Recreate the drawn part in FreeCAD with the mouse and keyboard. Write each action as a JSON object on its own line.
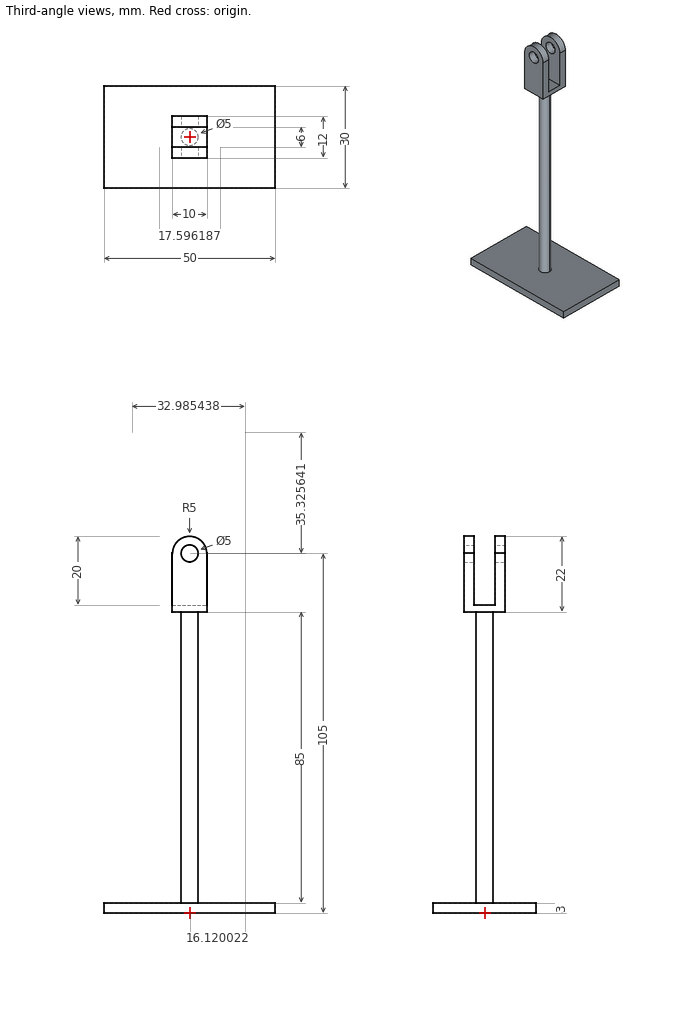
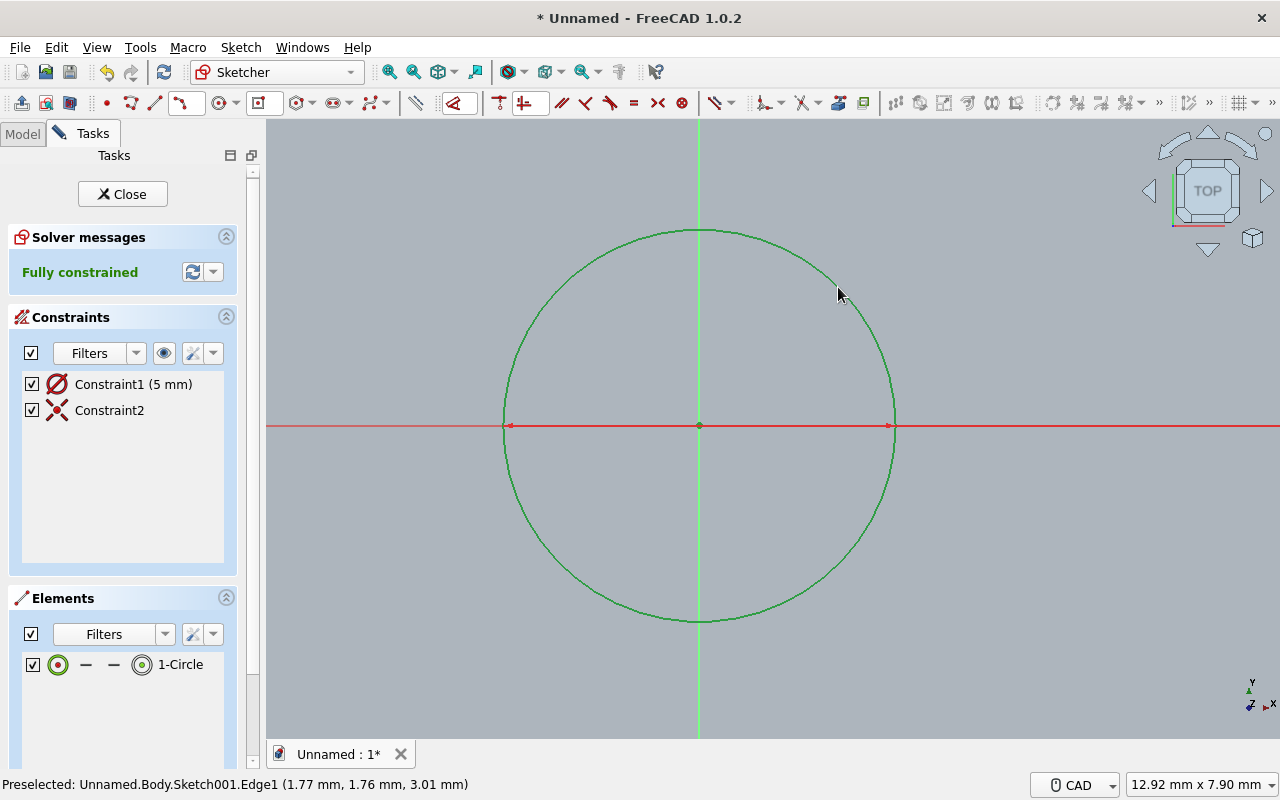
{"action": "left_click", "coordinate": [123, 194]}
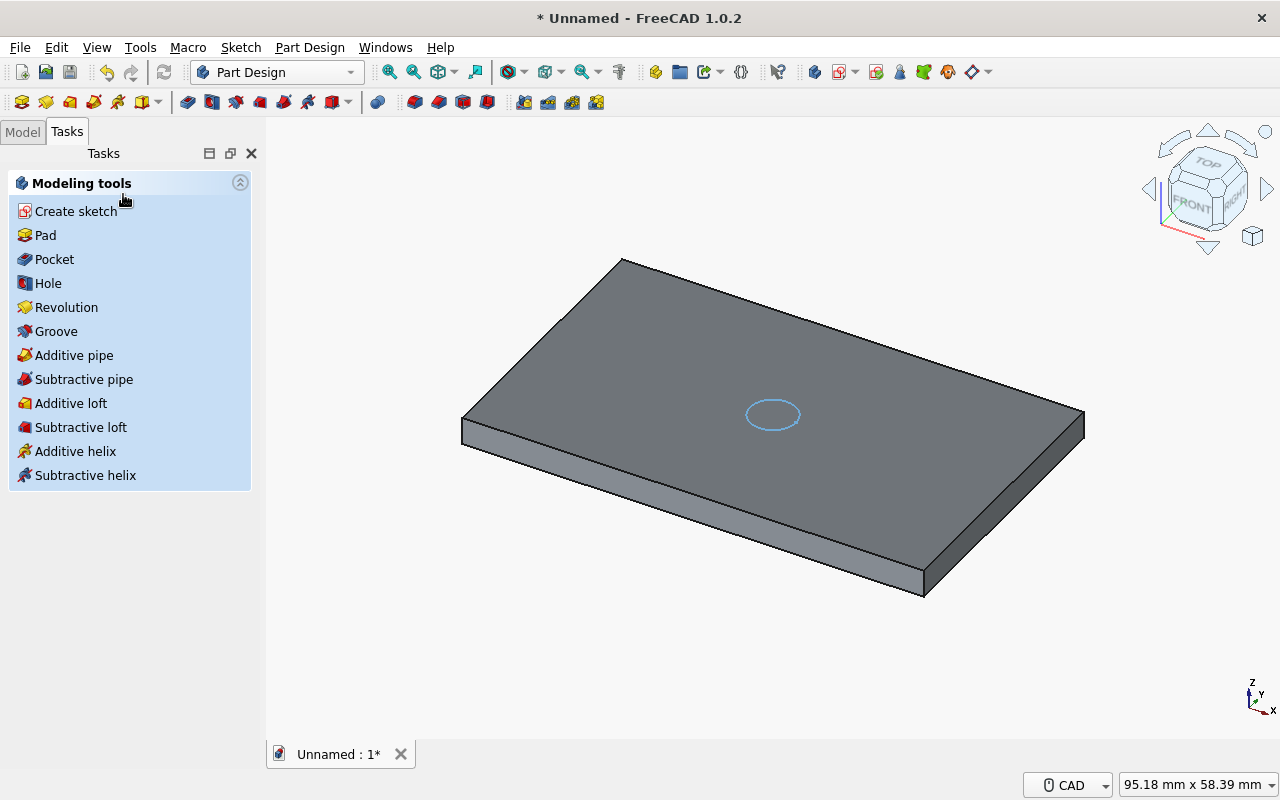
{"action": "left_click", "coordinate": [22, 102]}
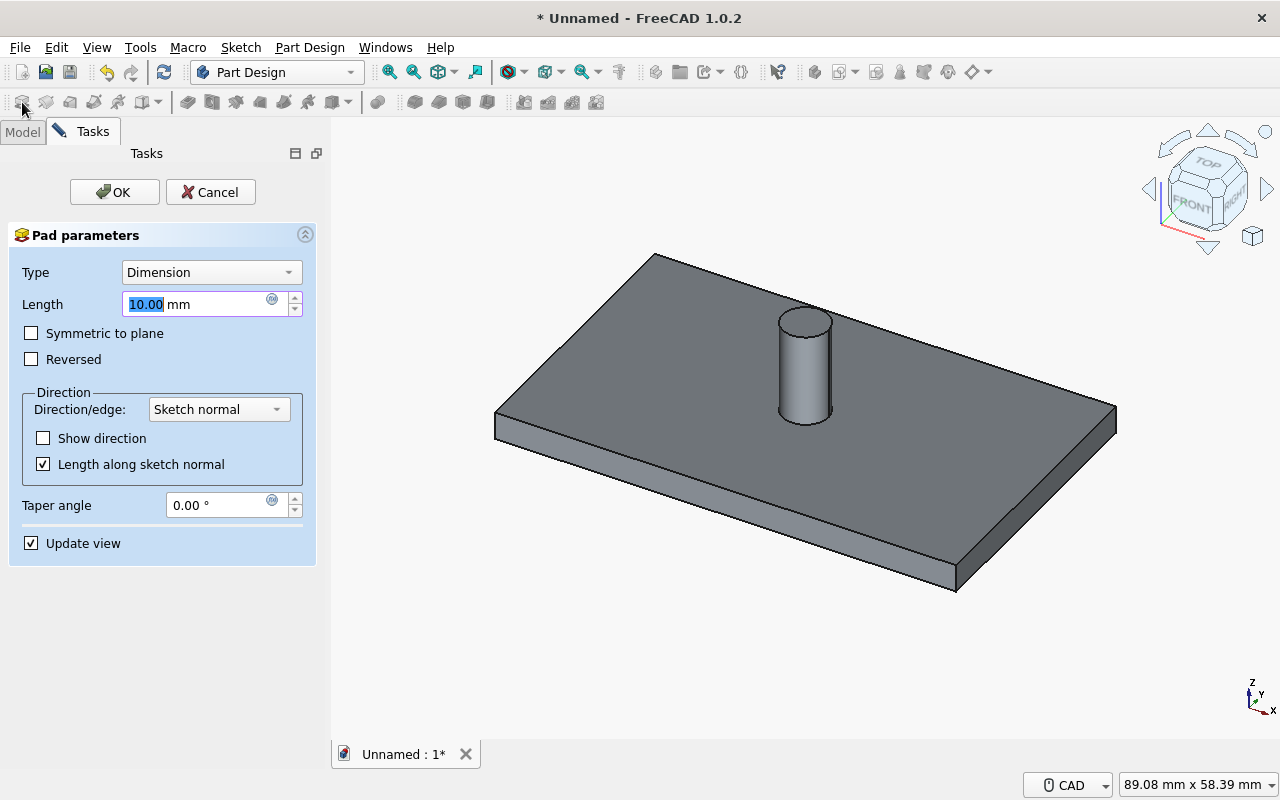
{"action": "type", "text": "85"}
{"action": "key", "text": "Tab"}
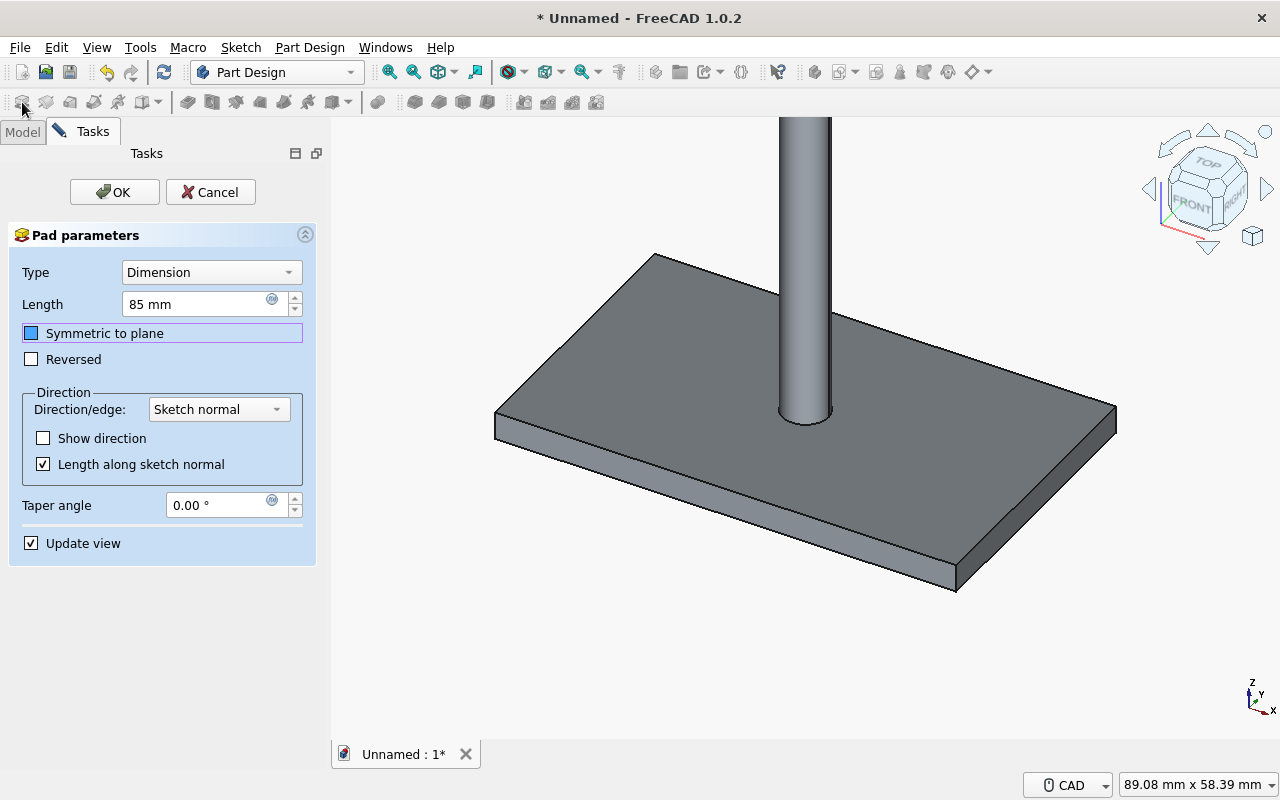
{"action": "left_click", "coordinate": [115, 192]}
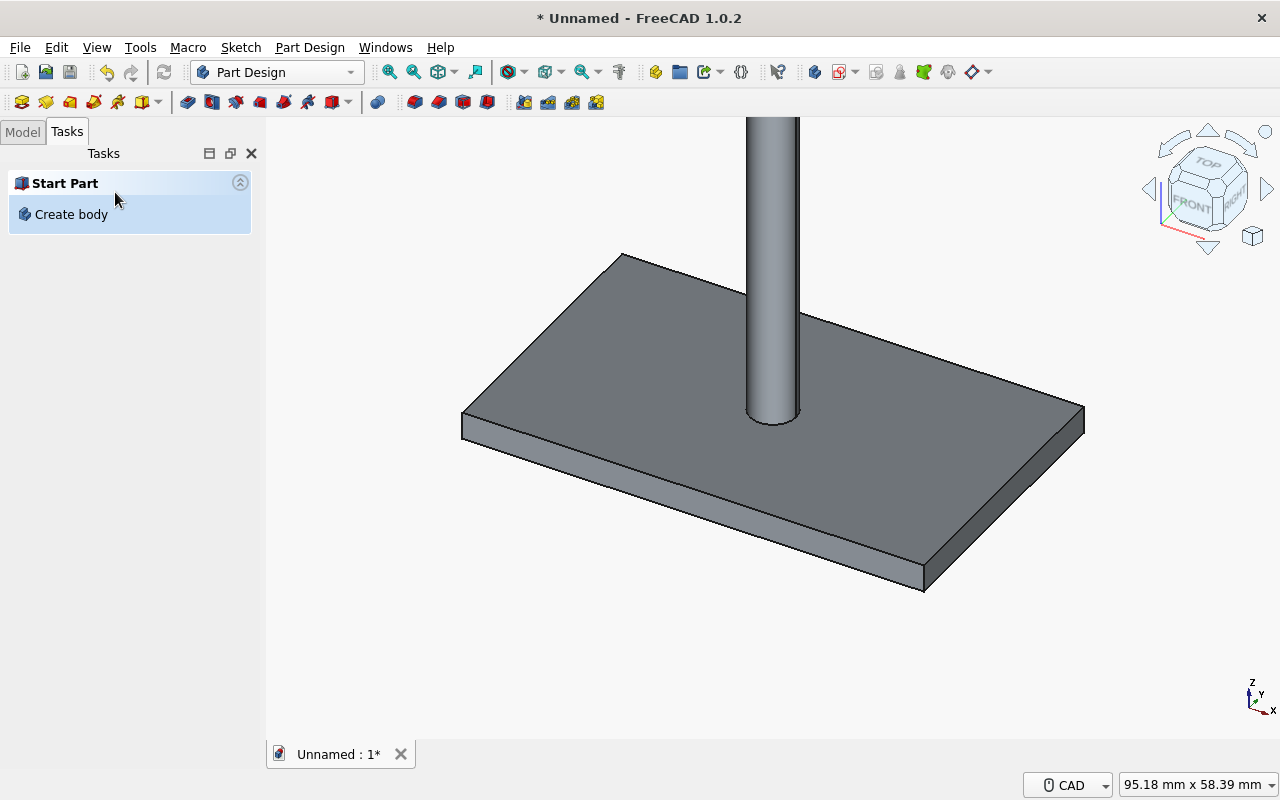
{"action": "left_click", "coordinate": [390, 72]}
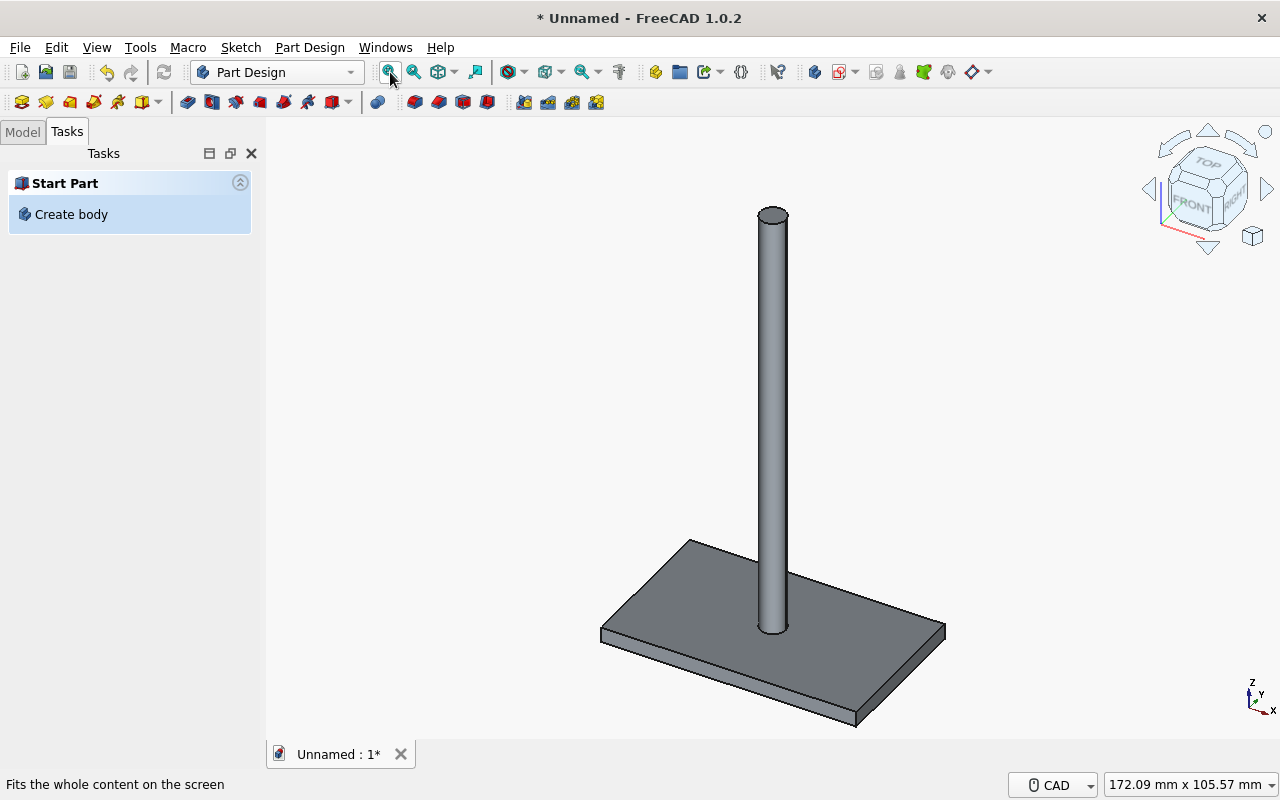
{"action": "left_click", "coordinate": [769, 213]}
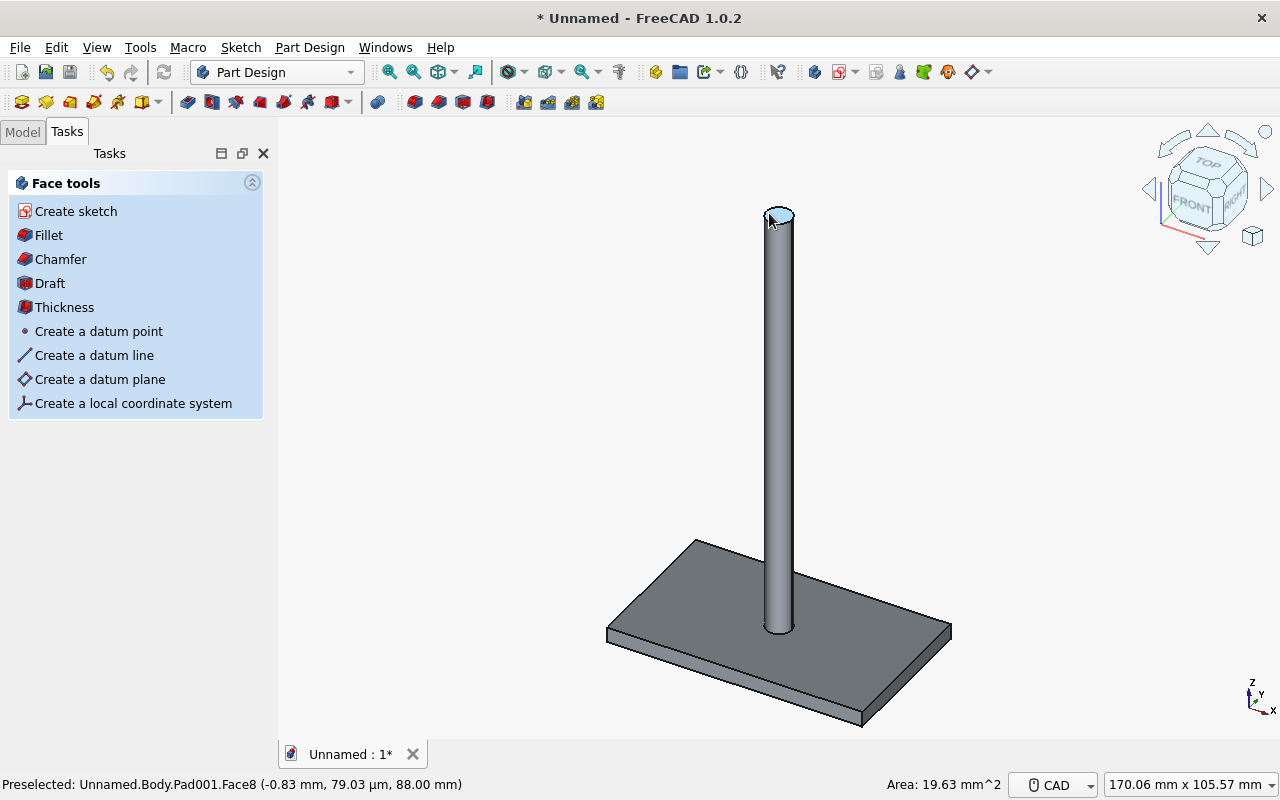
{"action": "left_click", "coordinate": [840, 72]}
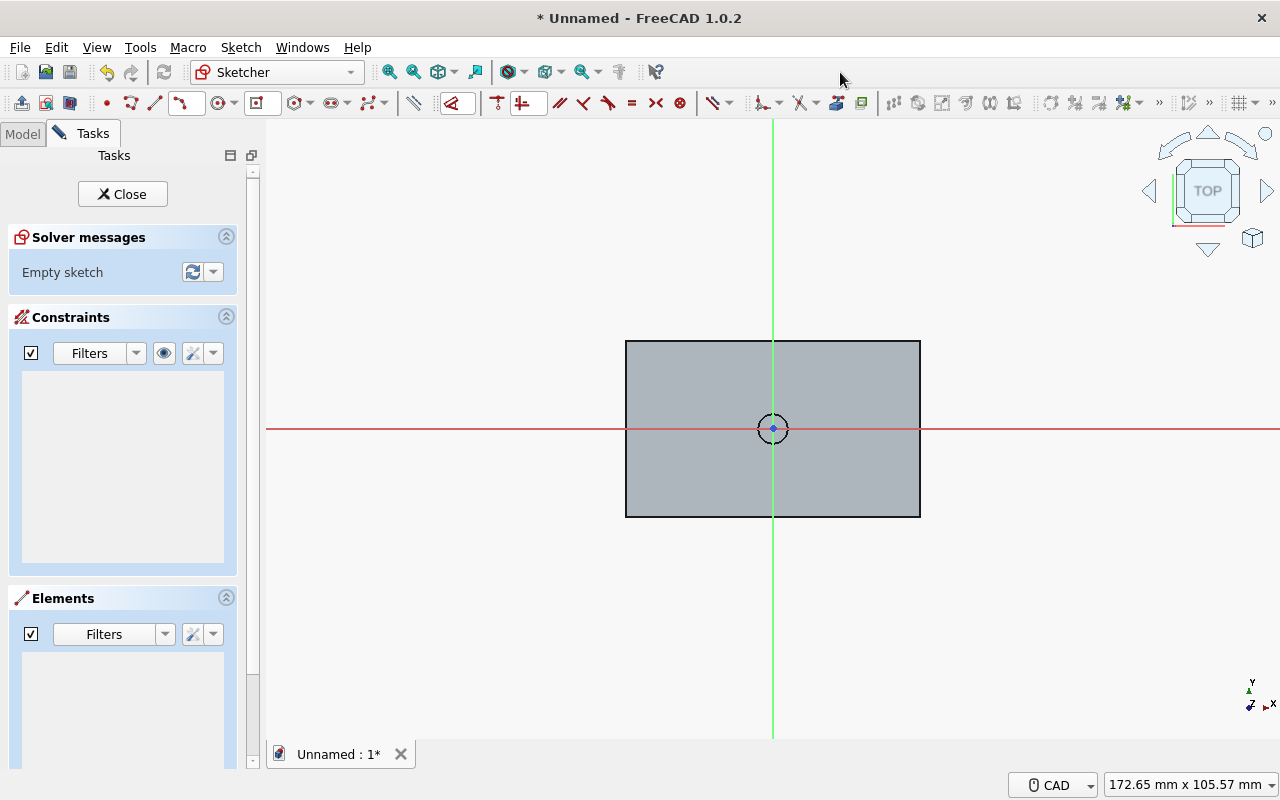
{"action": "scroll", "coordinate": [787, 429], "scroll_direction": "up", "scroll_amount": 9}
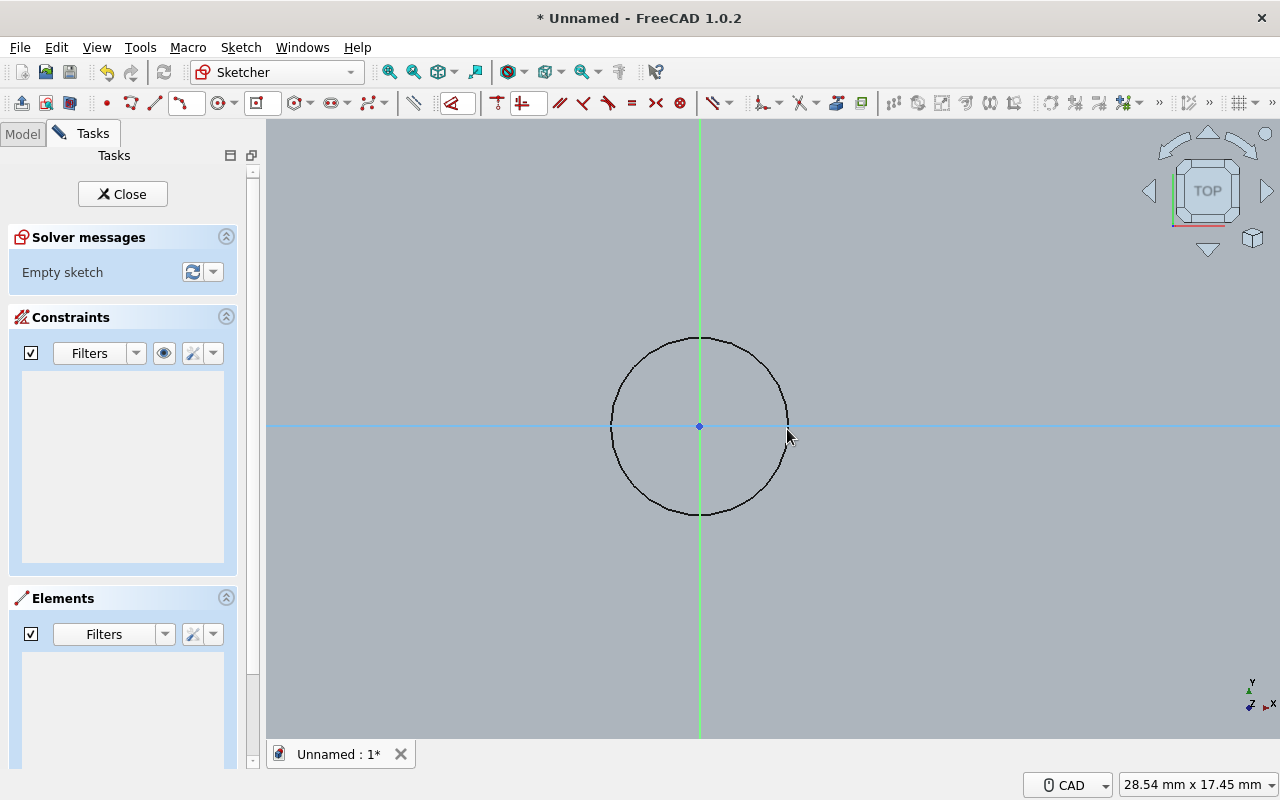
{"action": "left_click", "coordinate": [256, 104]}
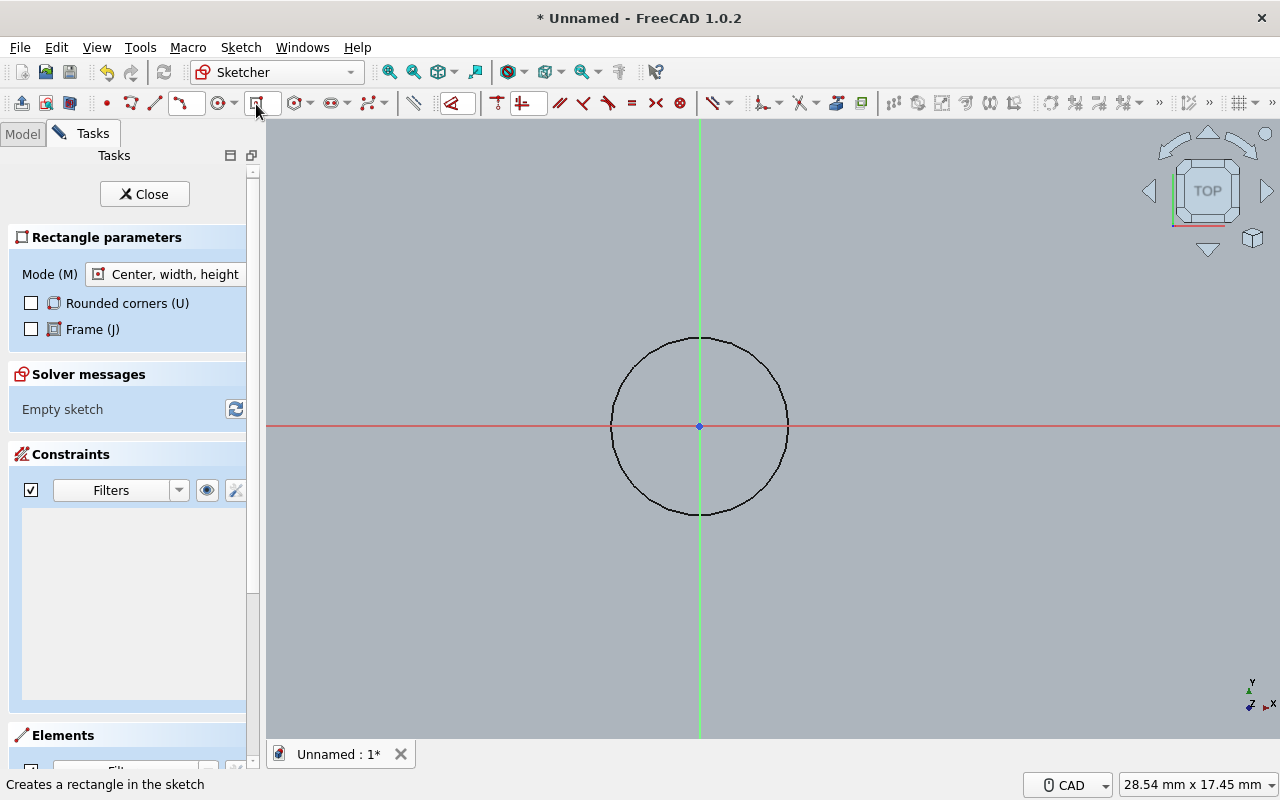
{"action": "left_click", "coordinate": [700, 426]}
{"action": "mouse_move", "coordinate": [877, 213]}